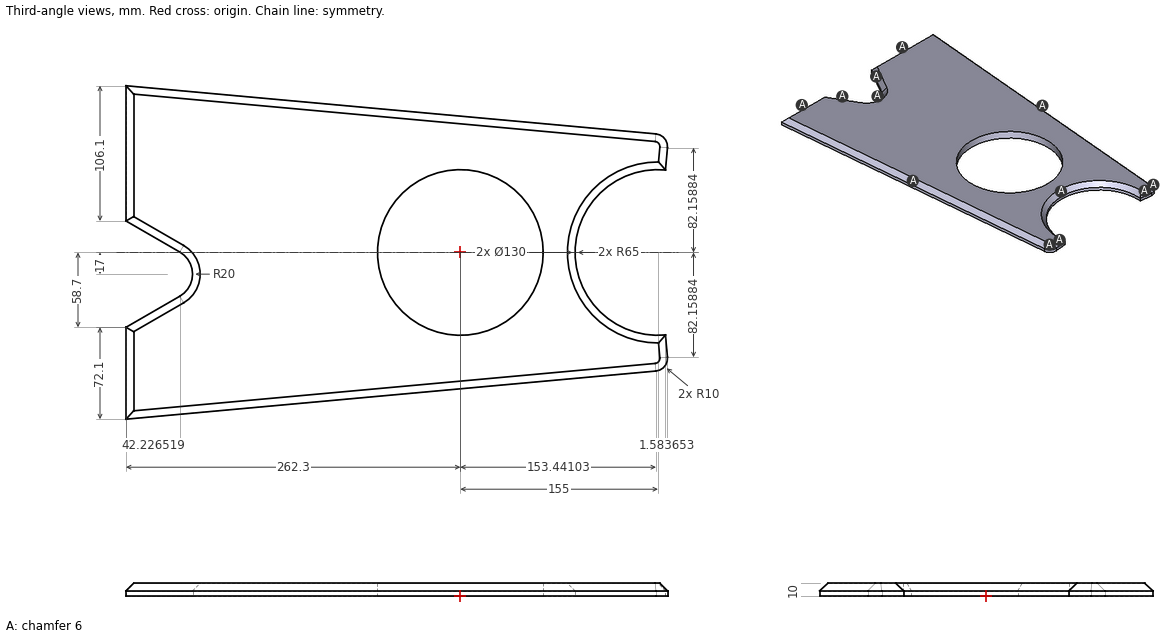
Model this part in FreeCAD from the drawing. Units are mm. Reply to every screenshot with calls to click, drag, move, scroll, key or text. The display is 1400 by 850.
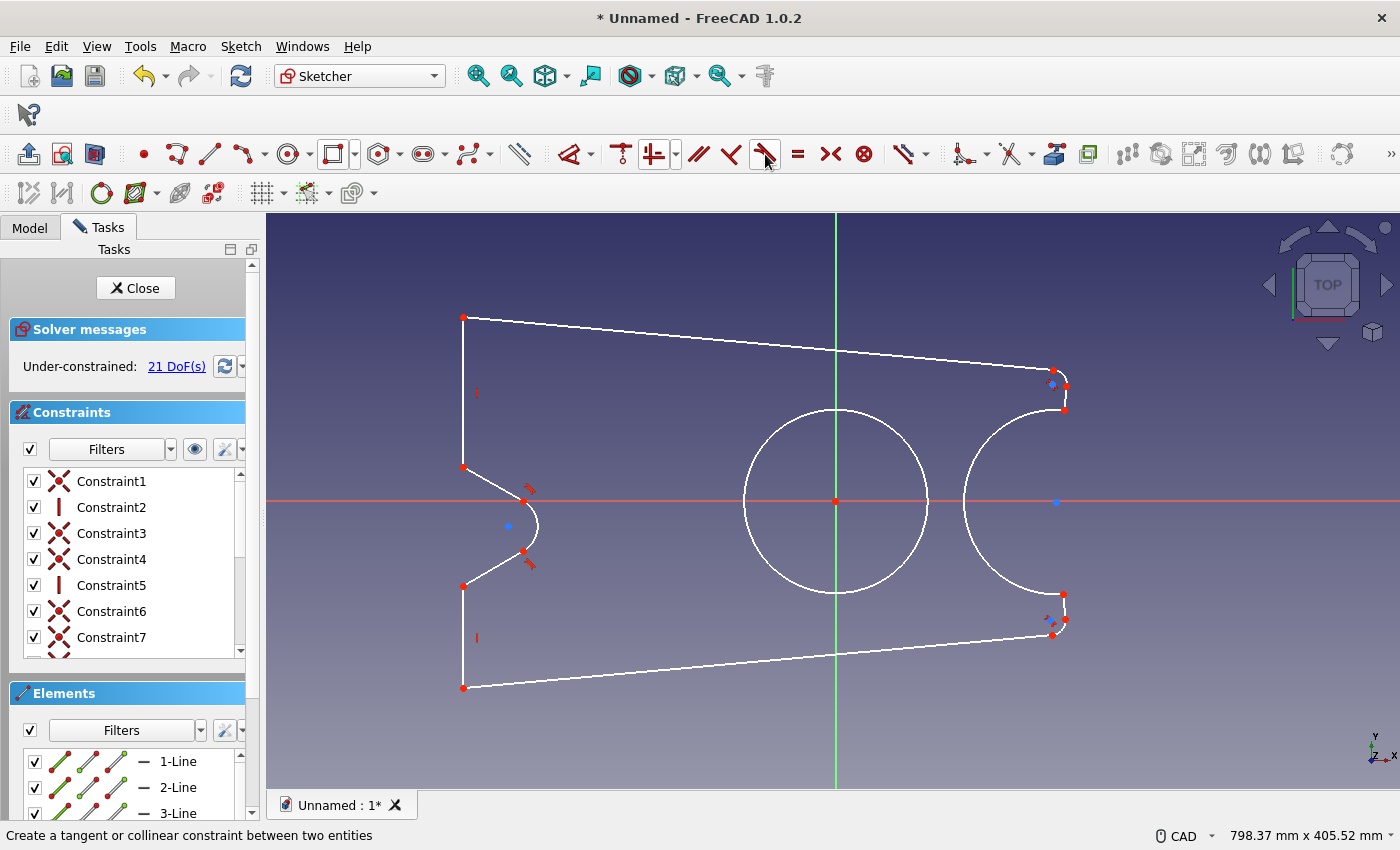
scroll(1062, 630, up, 2)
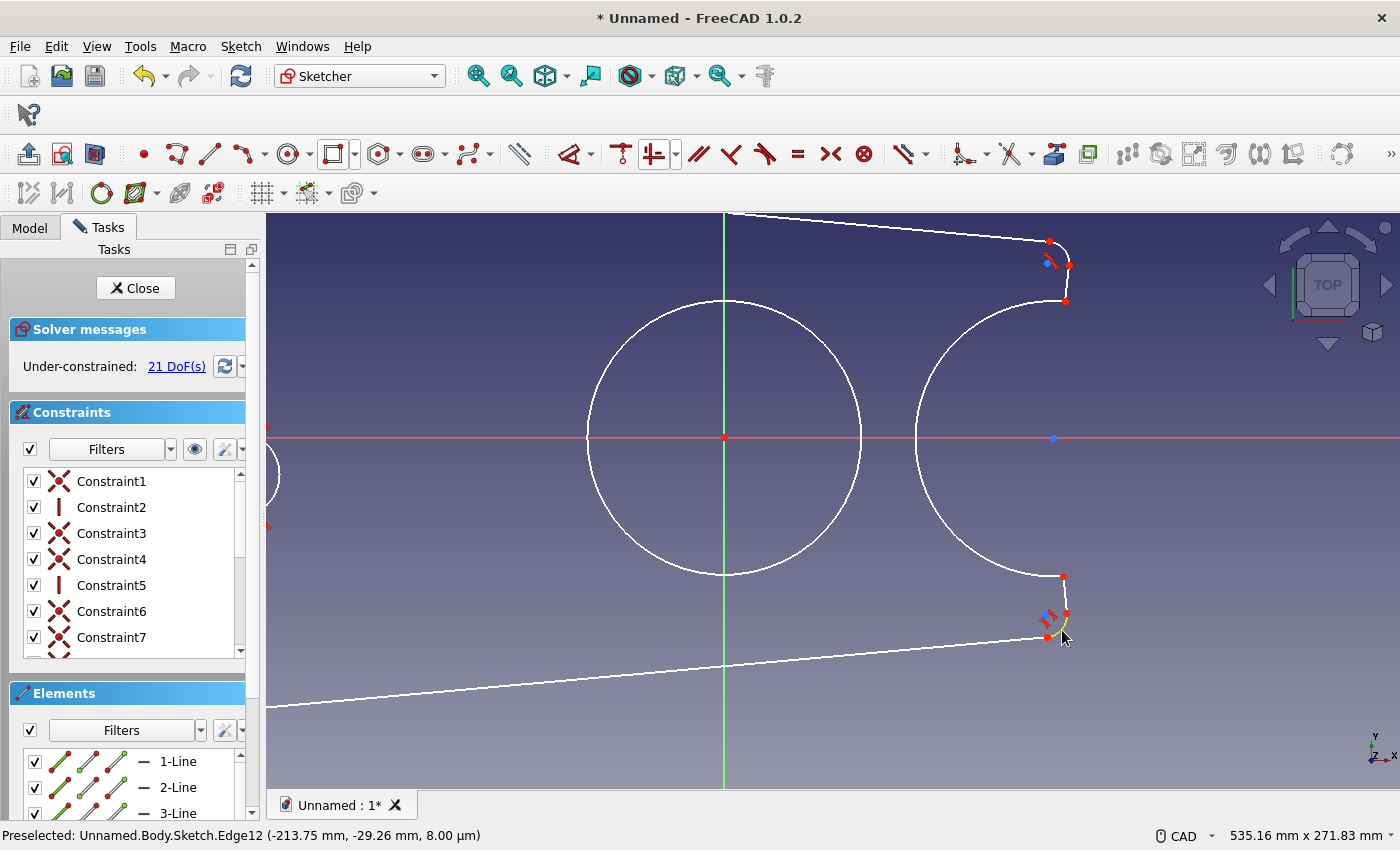
click(1062, 629)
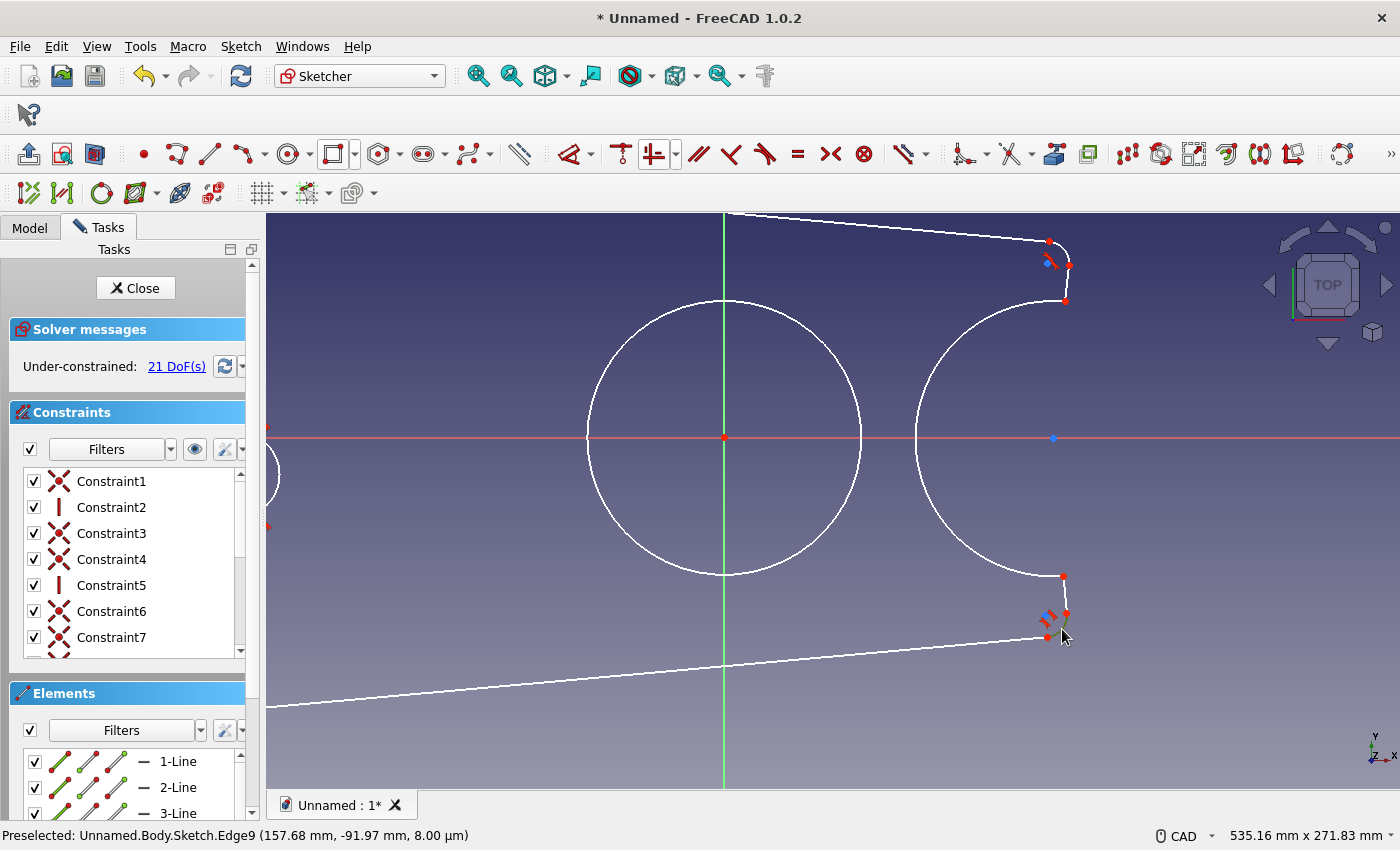
scroll(1068, 256, up, 2)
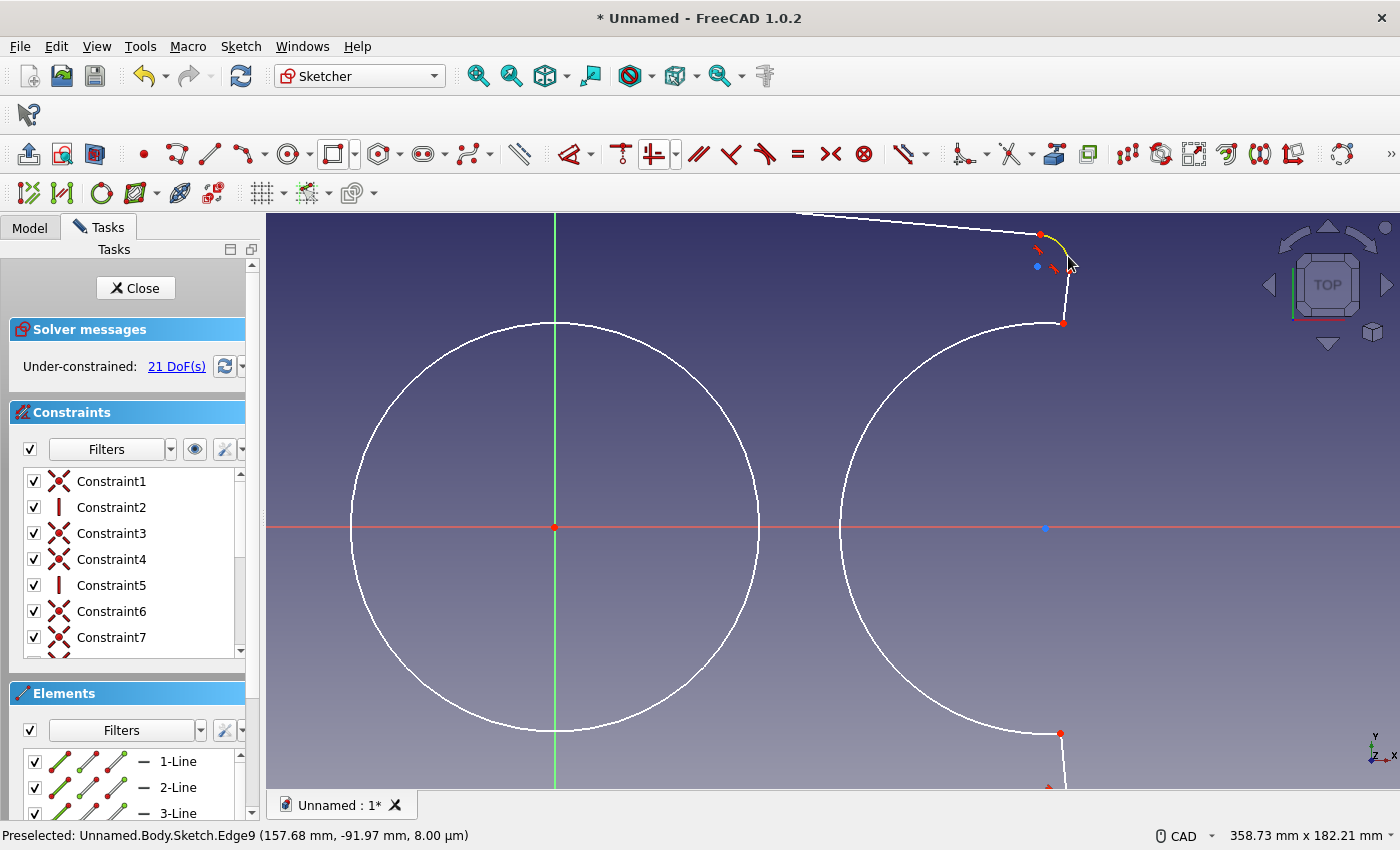
click(1067, 255)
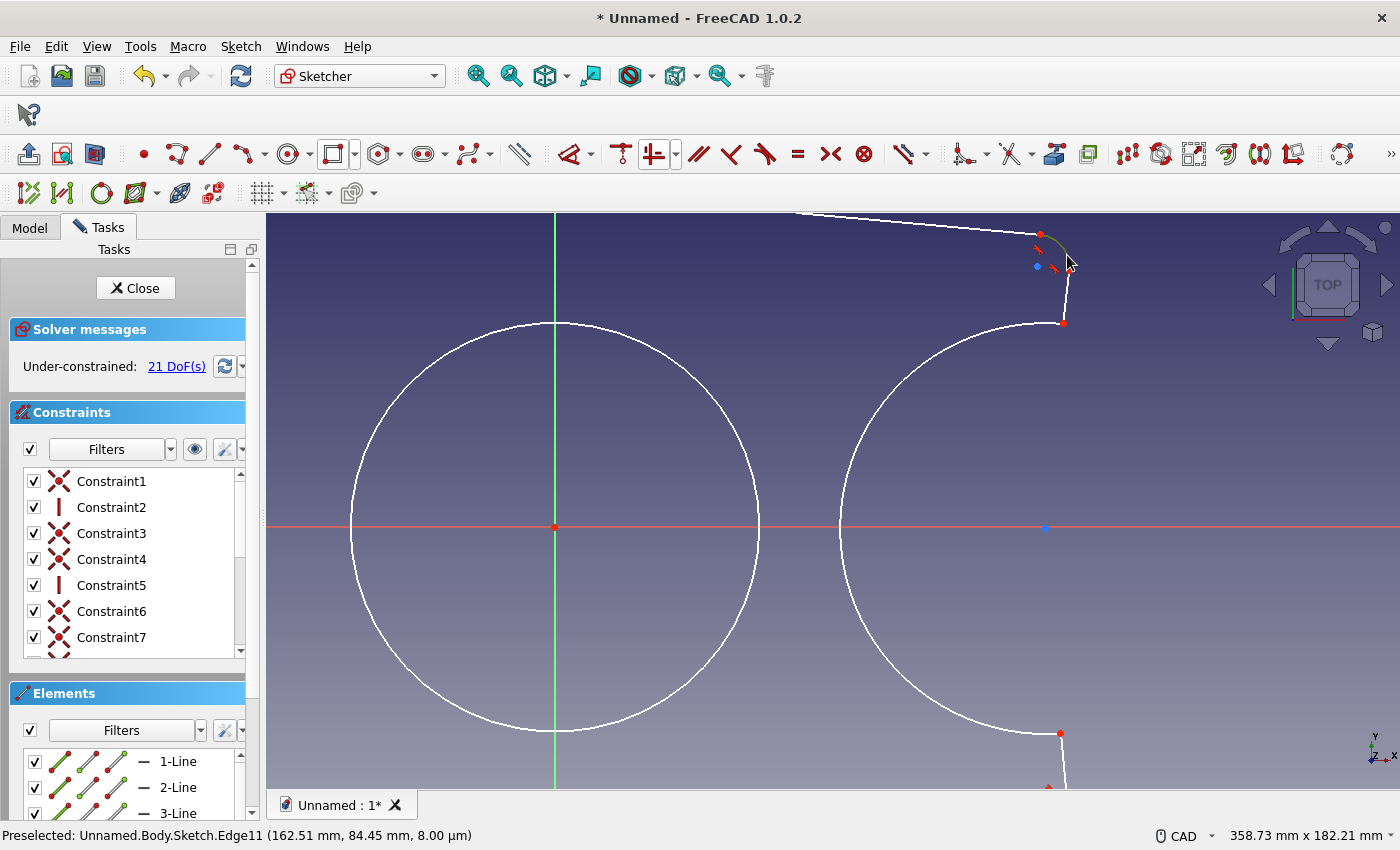
click(798, 154)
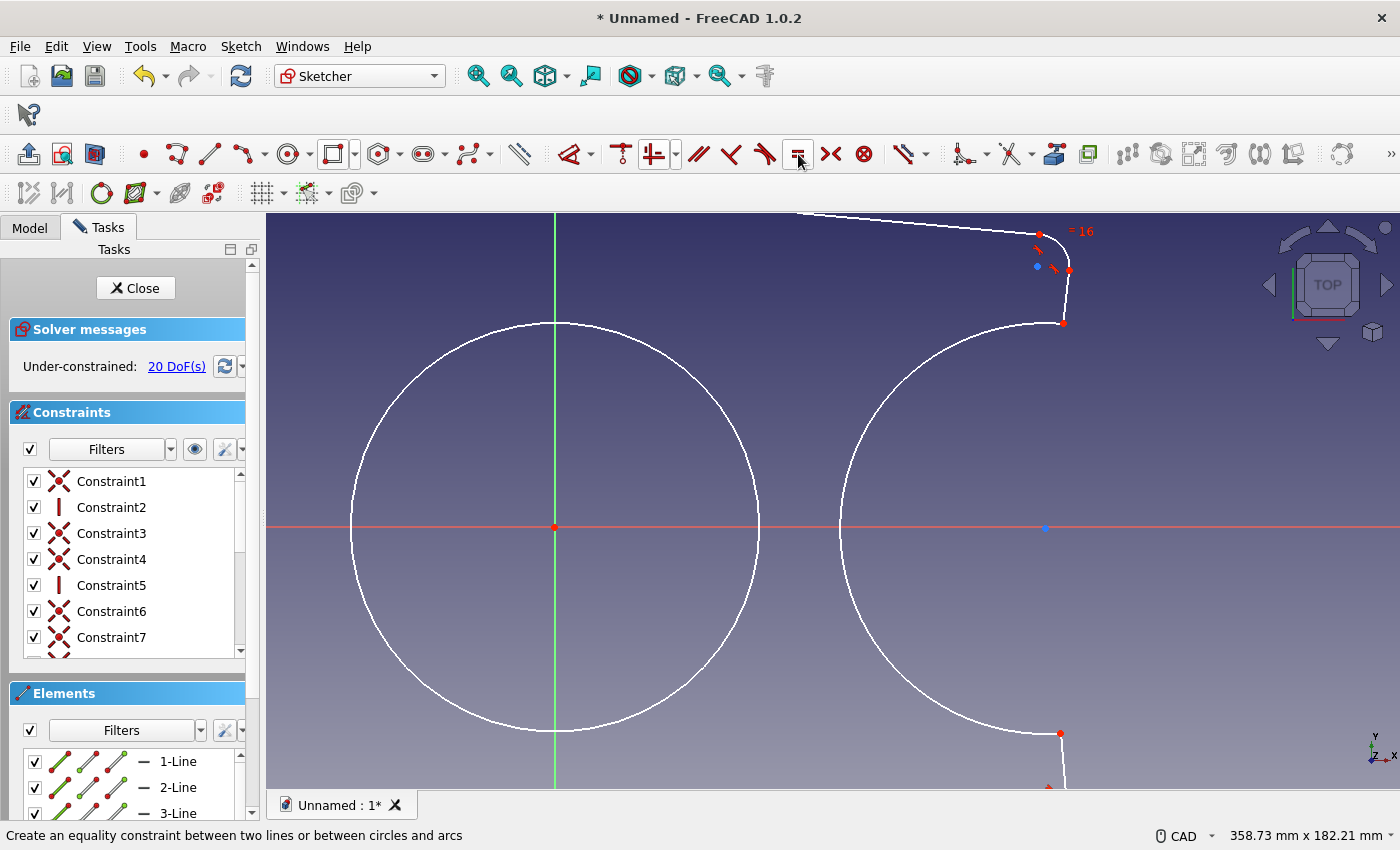
click(1046, 529)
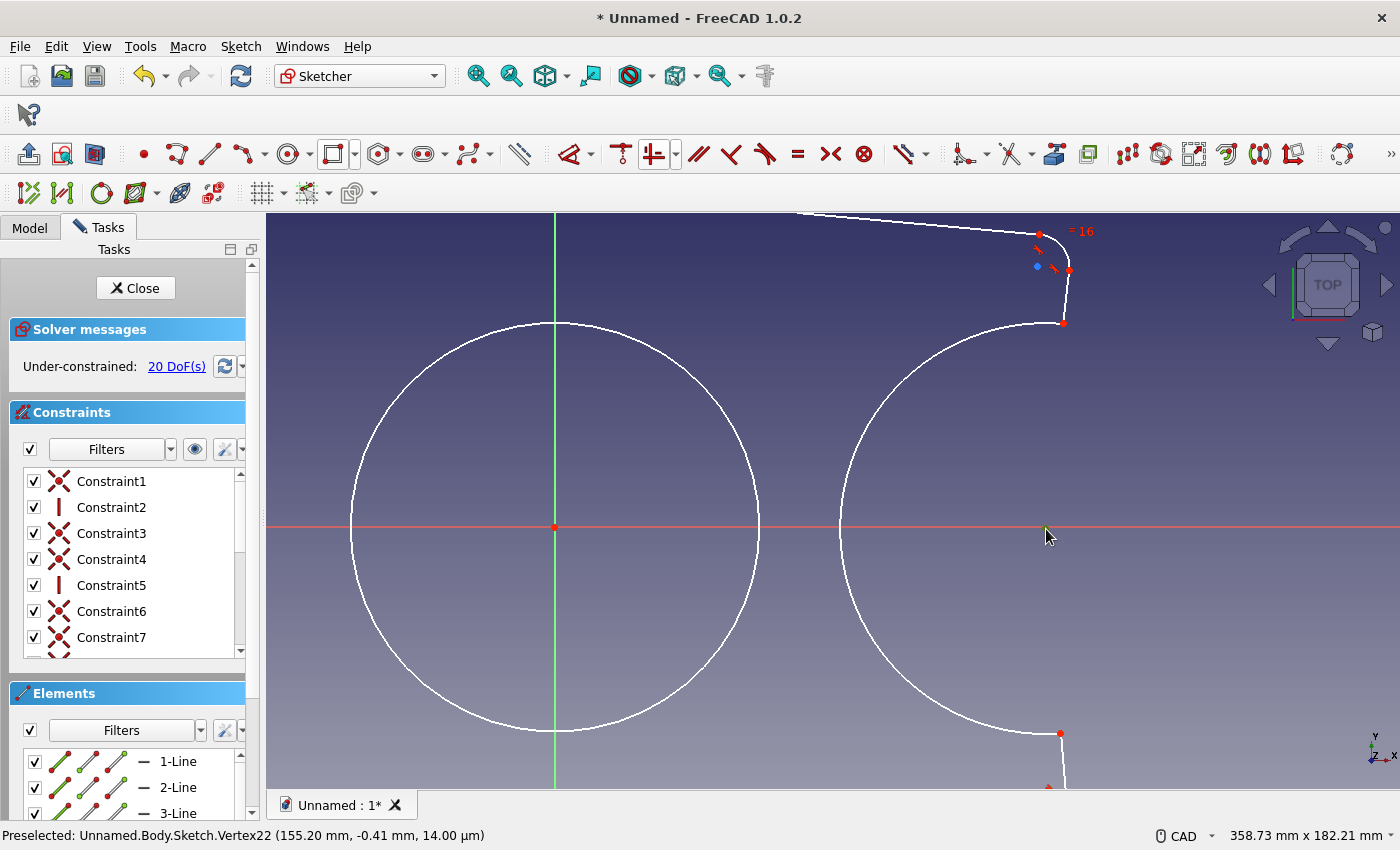
click(428, 527)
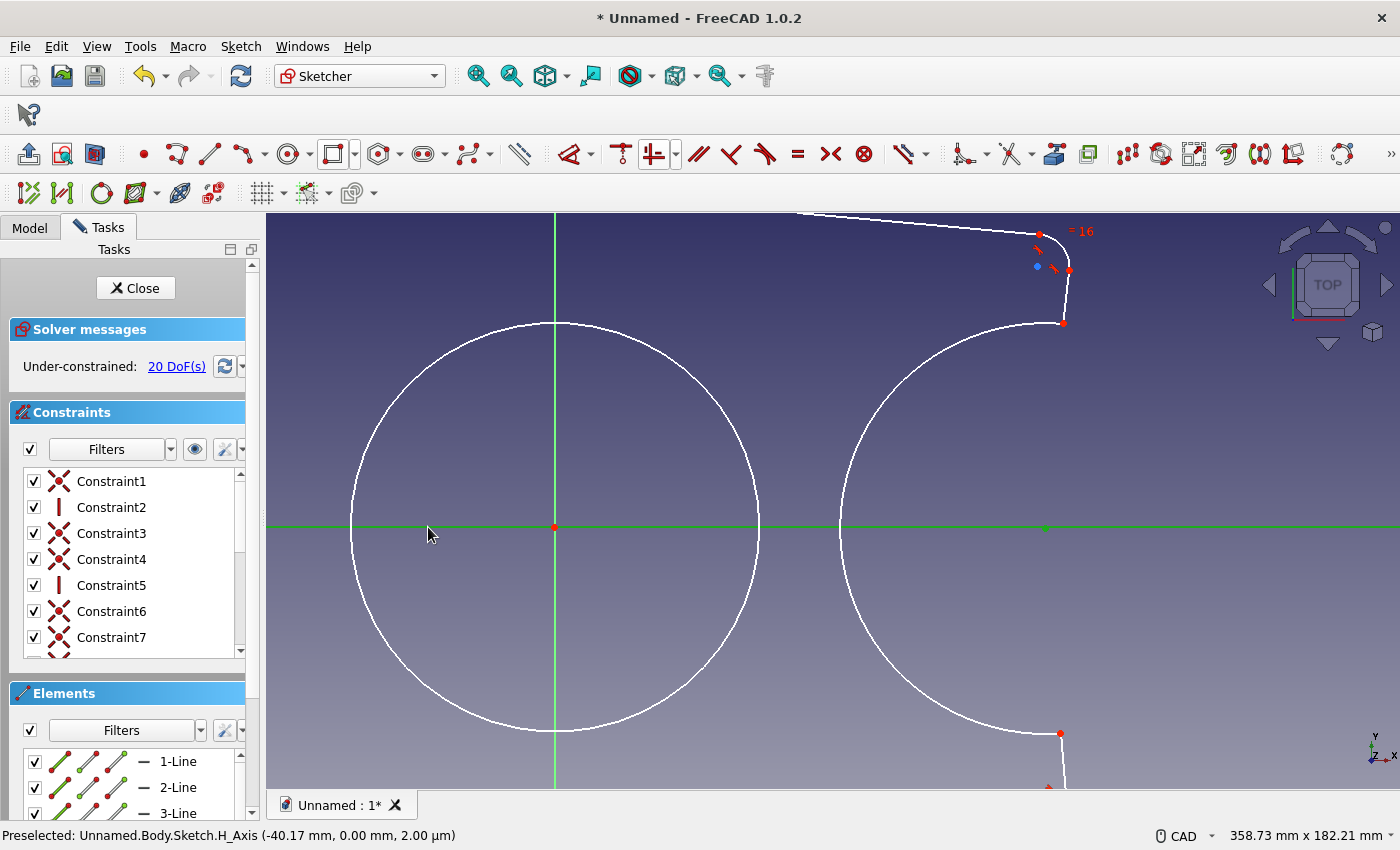
click(621, 154)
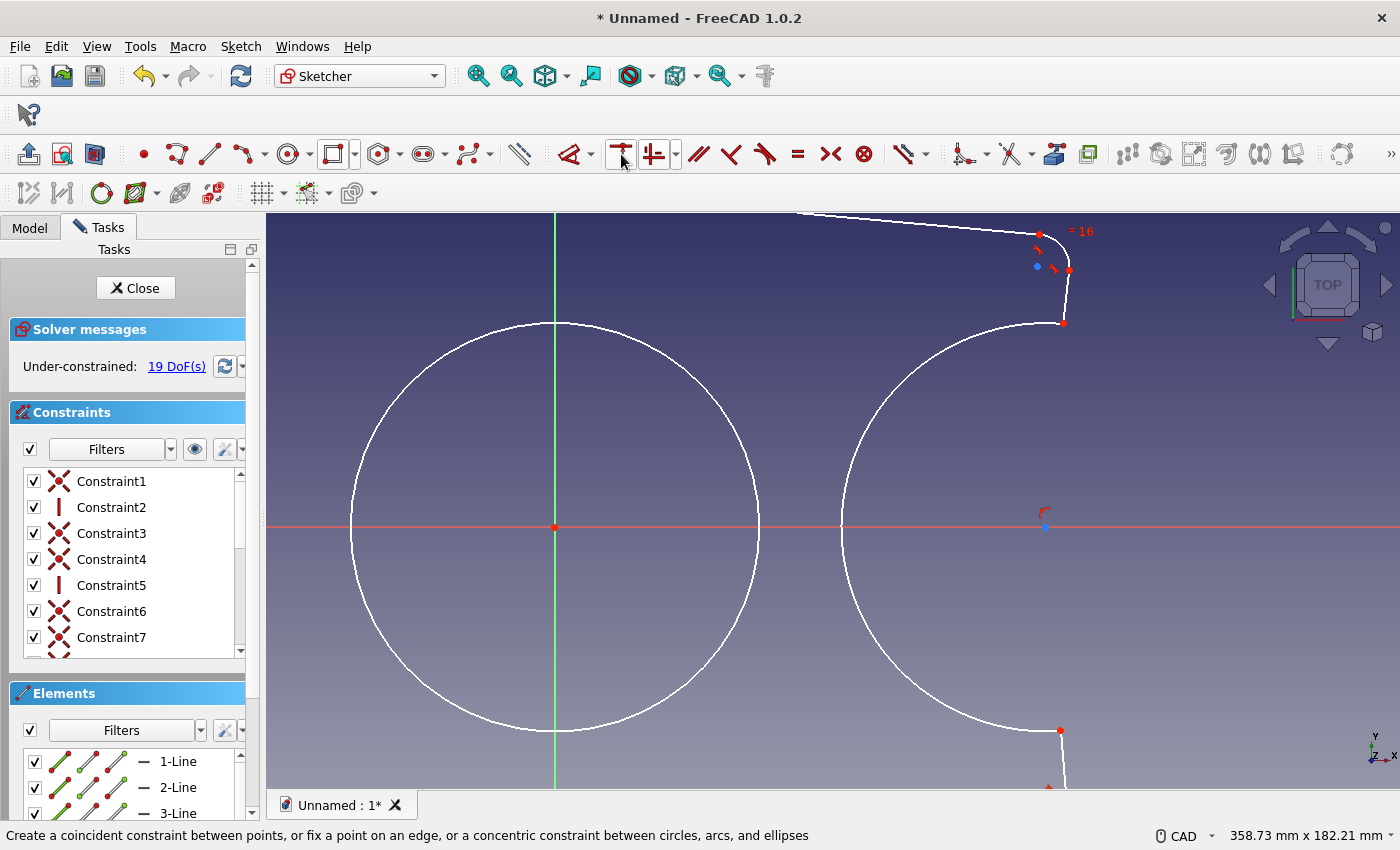
scroll(1064, 480, down, 4)